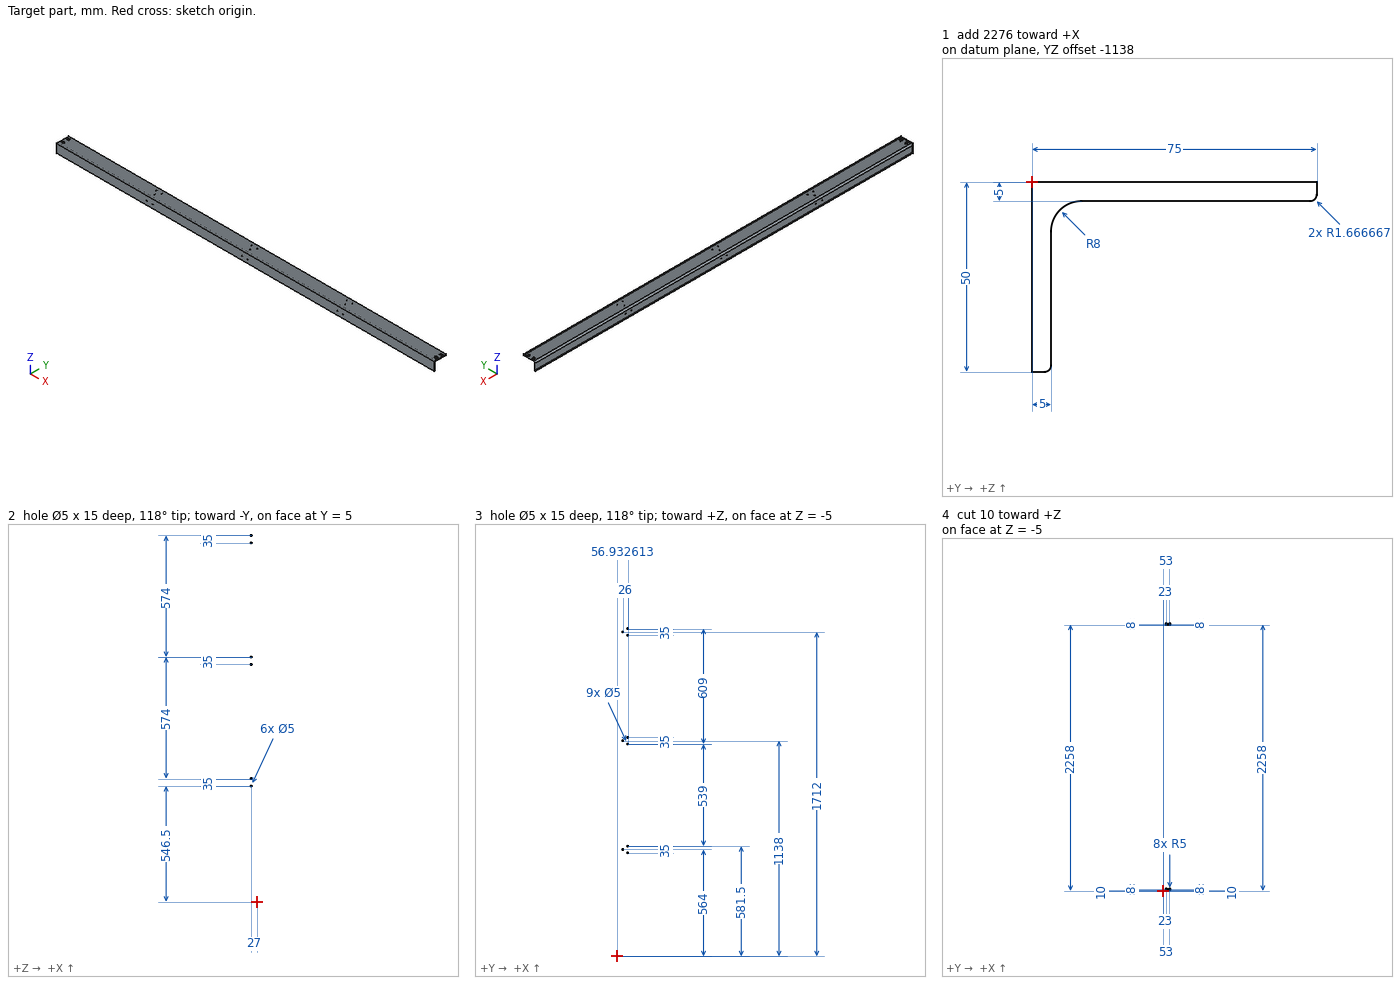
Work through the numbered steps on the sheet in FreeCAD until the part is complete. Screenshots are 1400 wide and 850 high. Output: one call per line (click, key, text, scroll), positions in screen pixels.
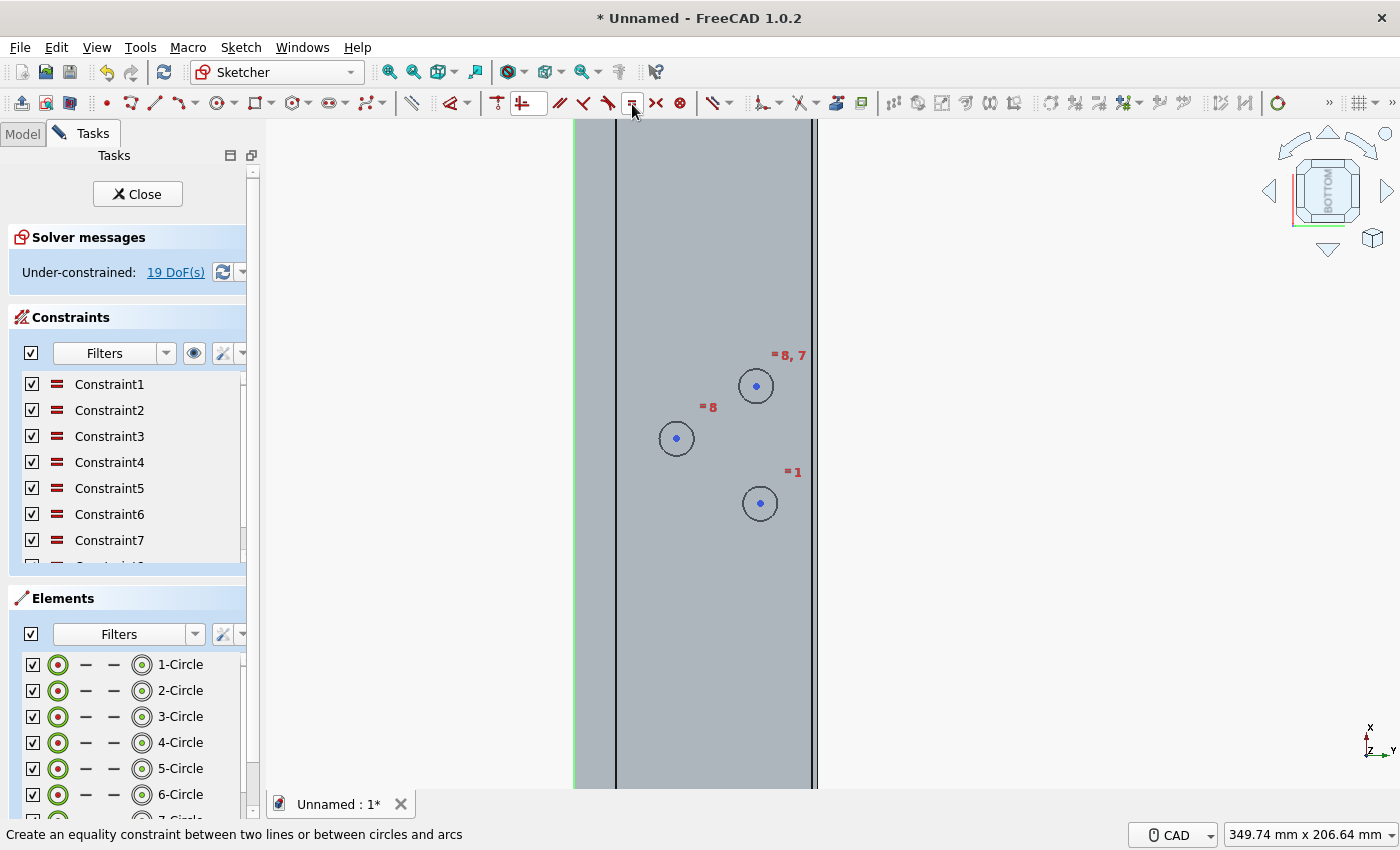
scroll(772, 385, down, 13)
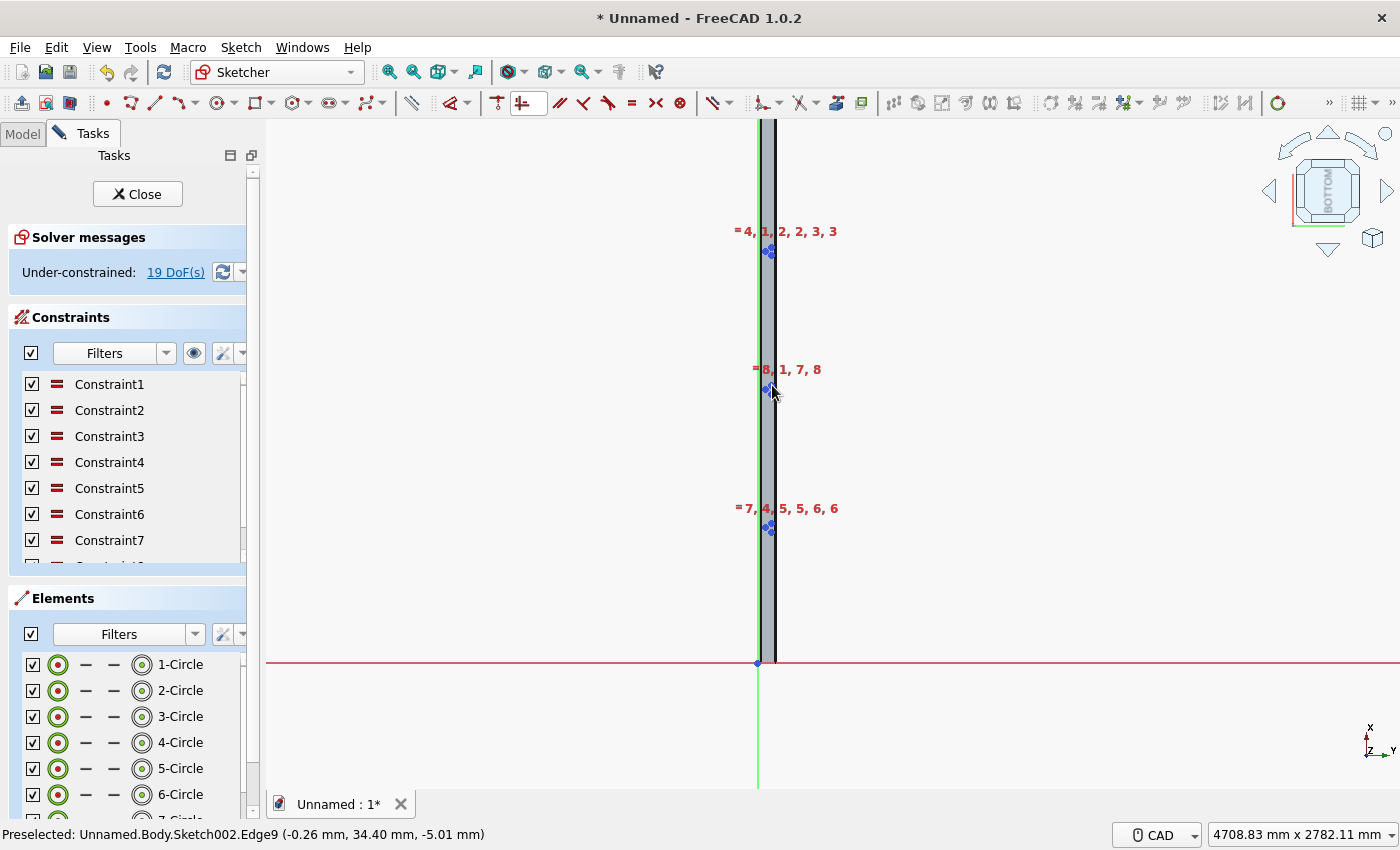
scroll(772, 394, up, 3)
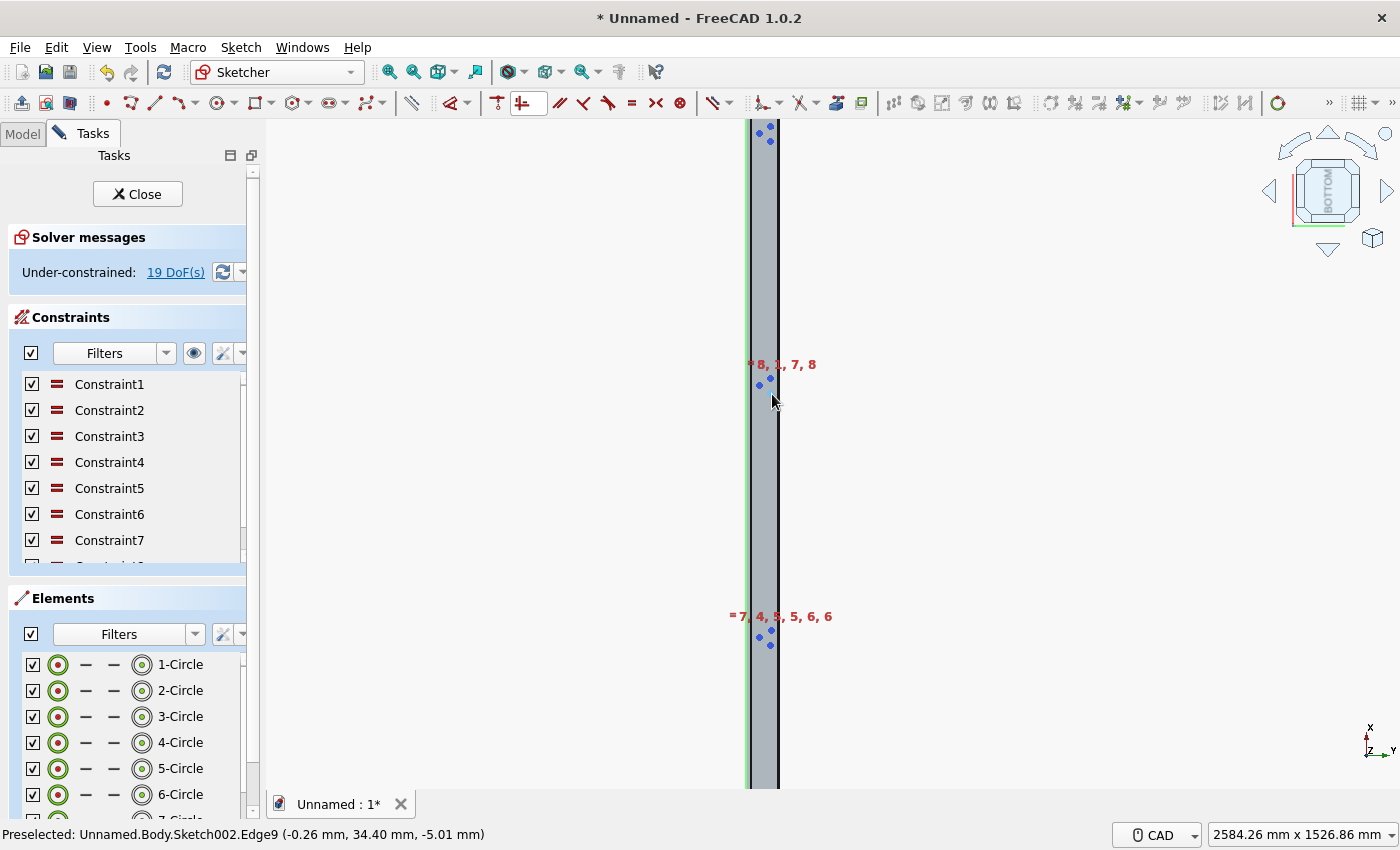
click(771, 394)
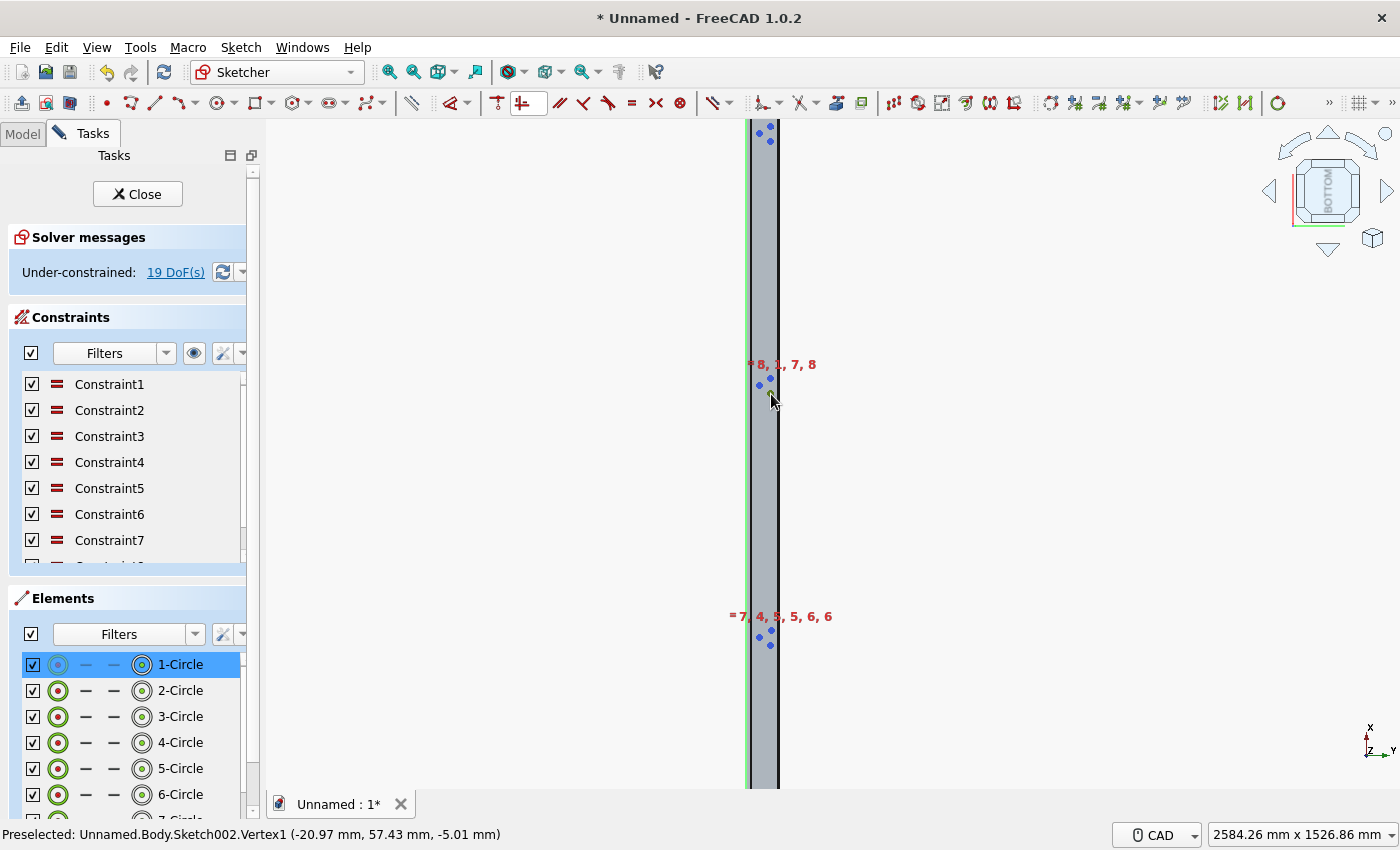
scroll(772, 393, down, 3)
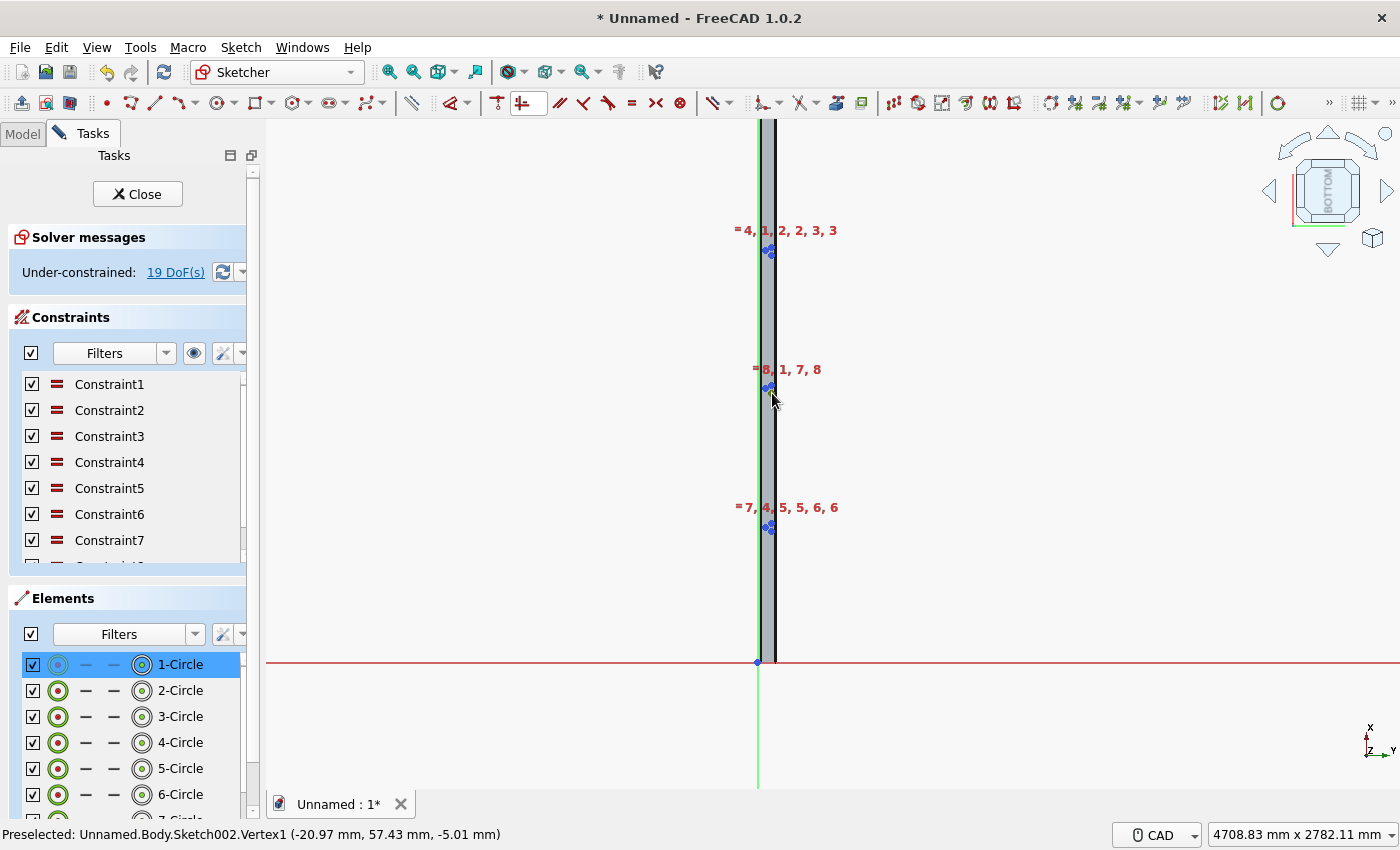
scroll(772, 247, up, 3)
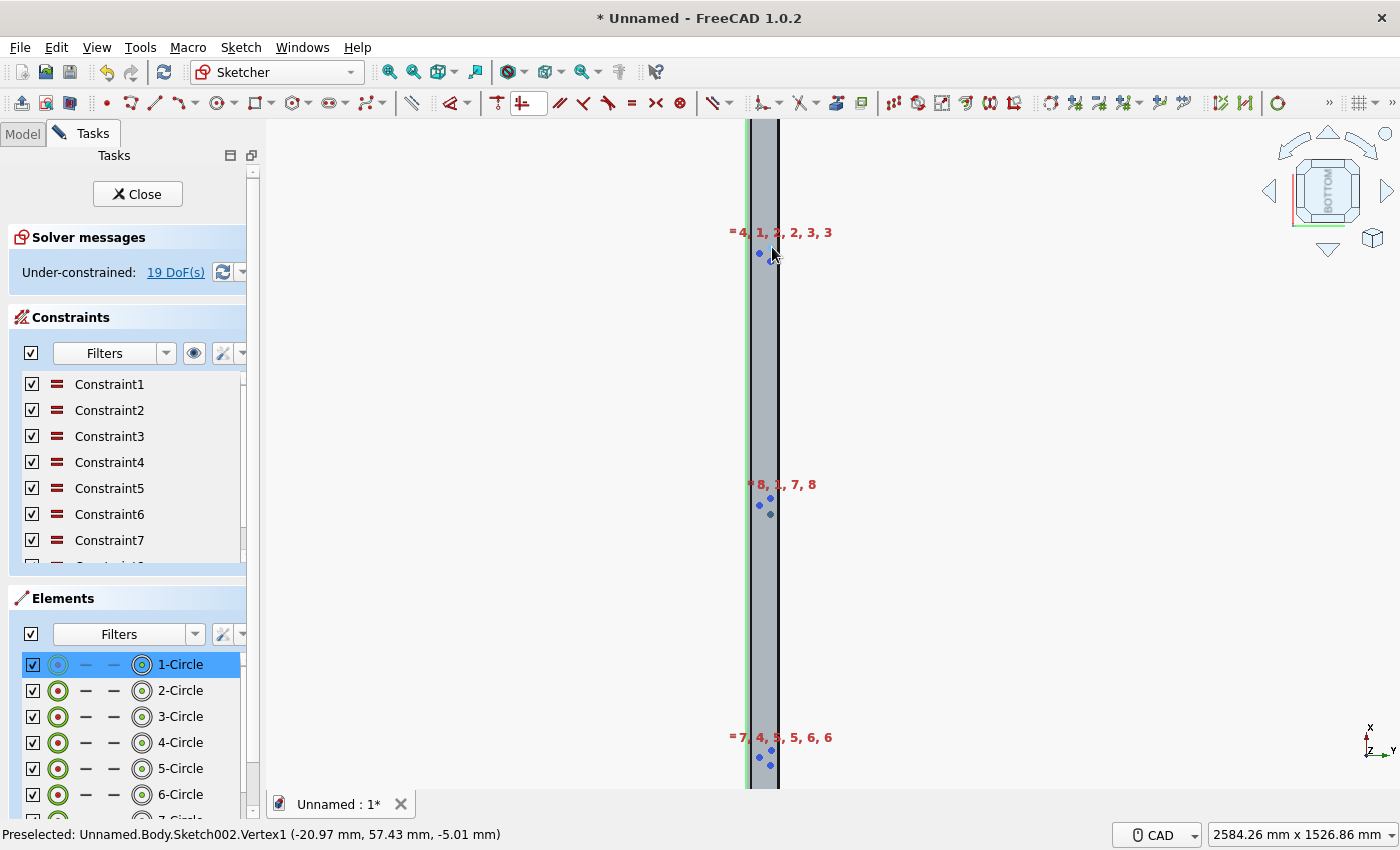
click(771, 247)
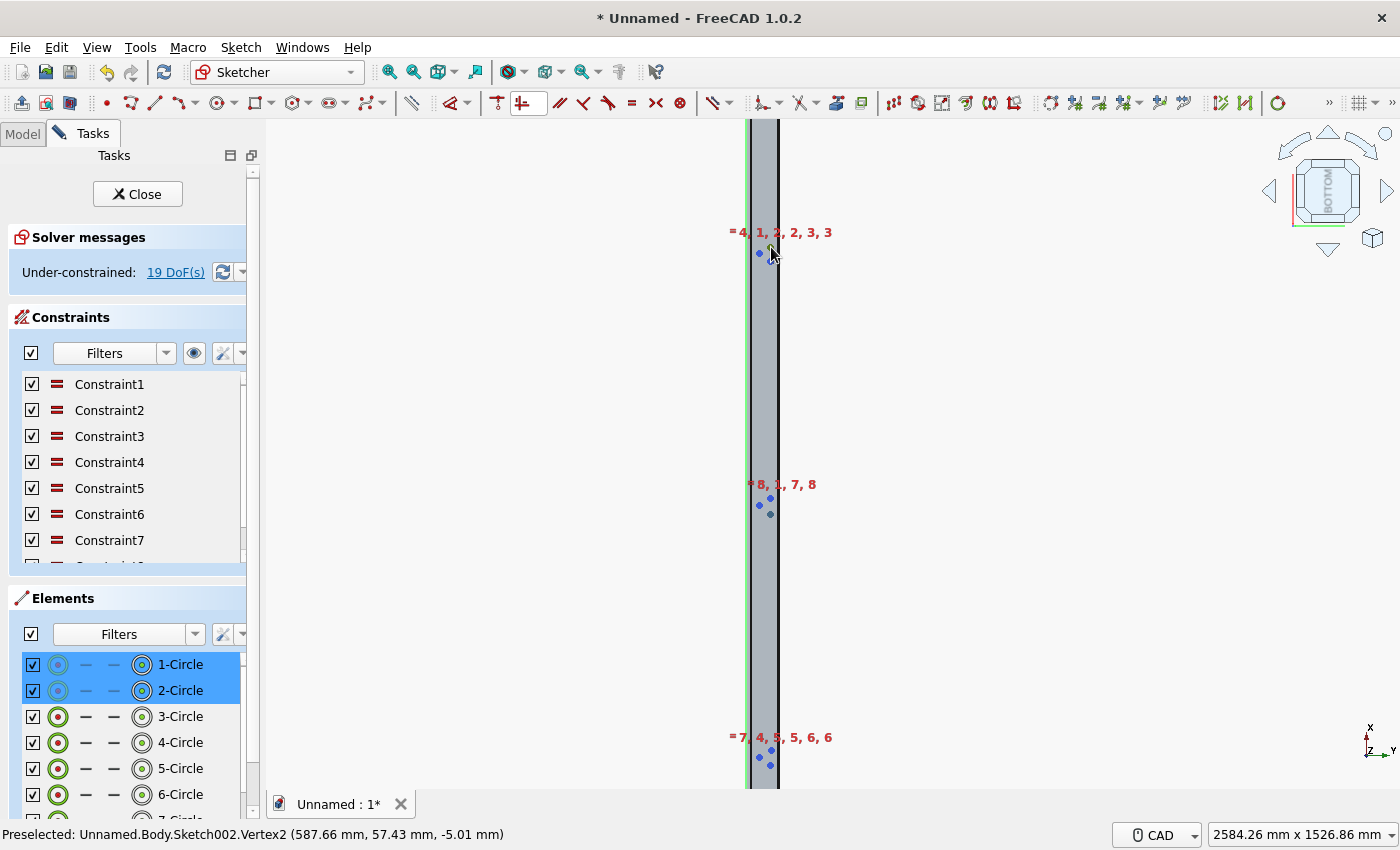
key(v)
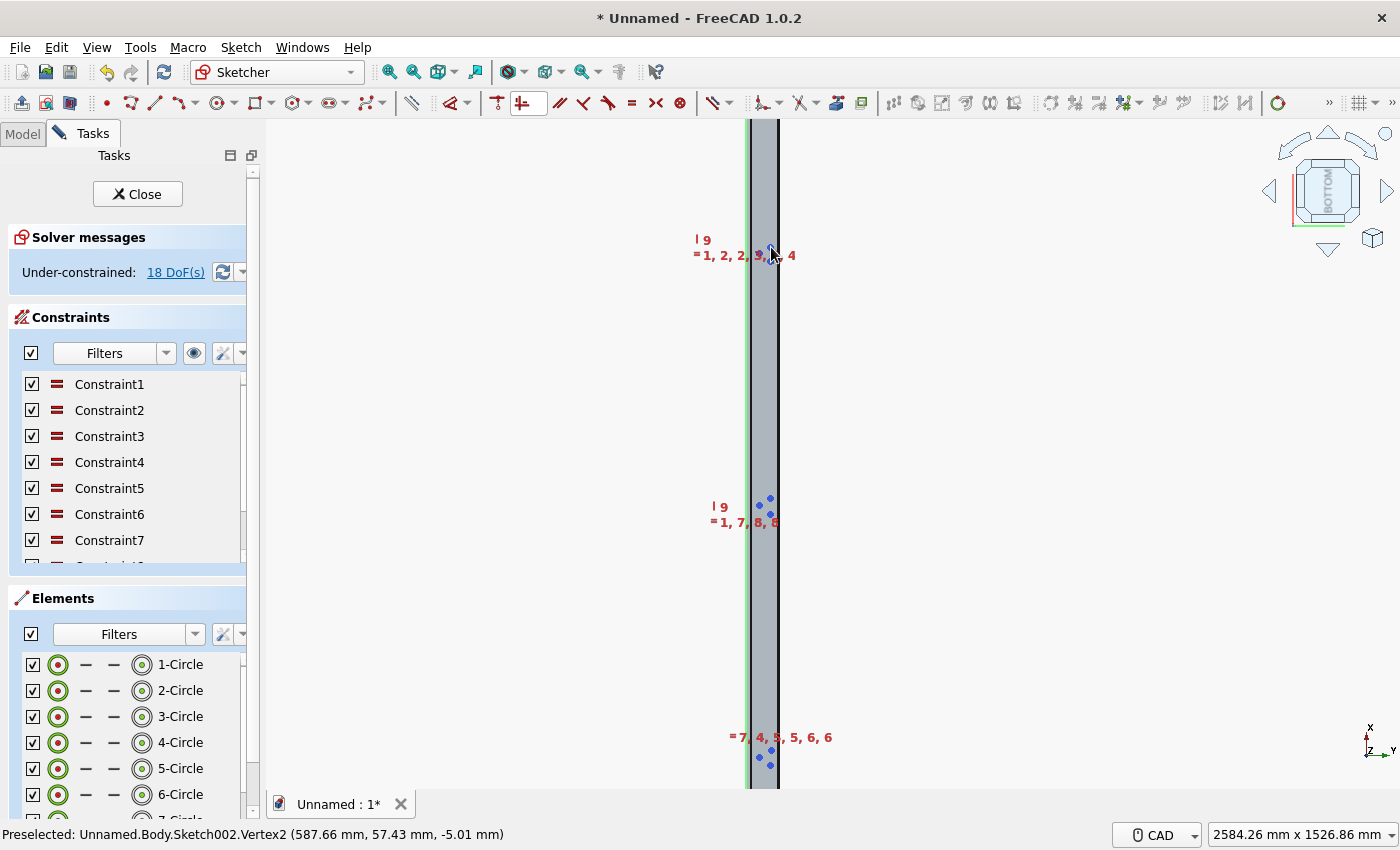
scroll(771, 247, up, 4)